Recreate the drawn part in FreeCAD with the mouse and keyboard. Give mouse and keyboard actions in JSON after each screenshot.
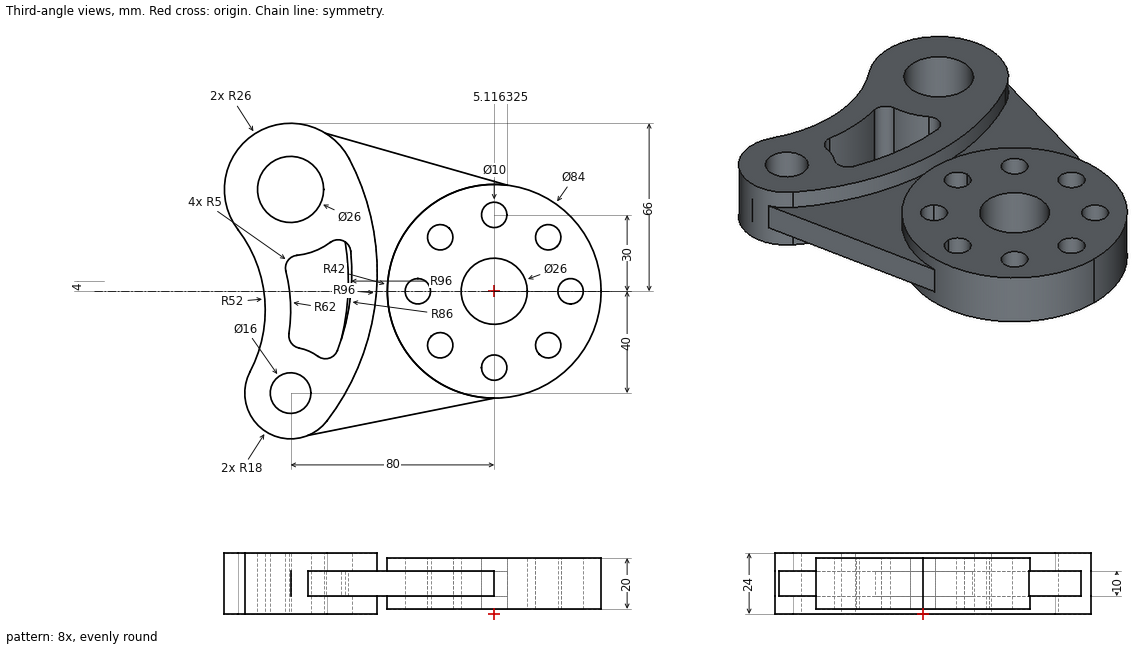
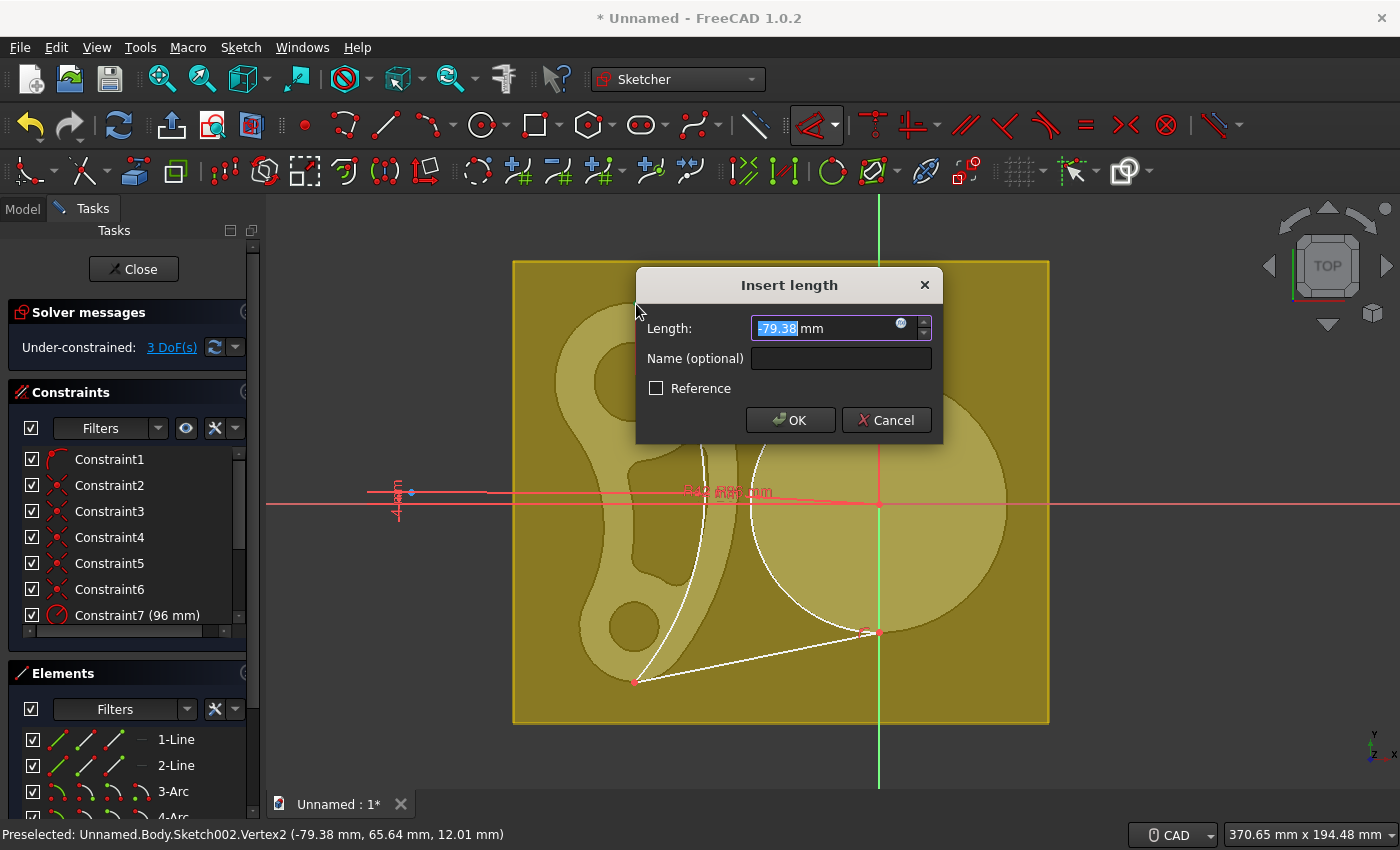
{"action": "type", "text": "-80"}
{"action": "key", "text": "Return"}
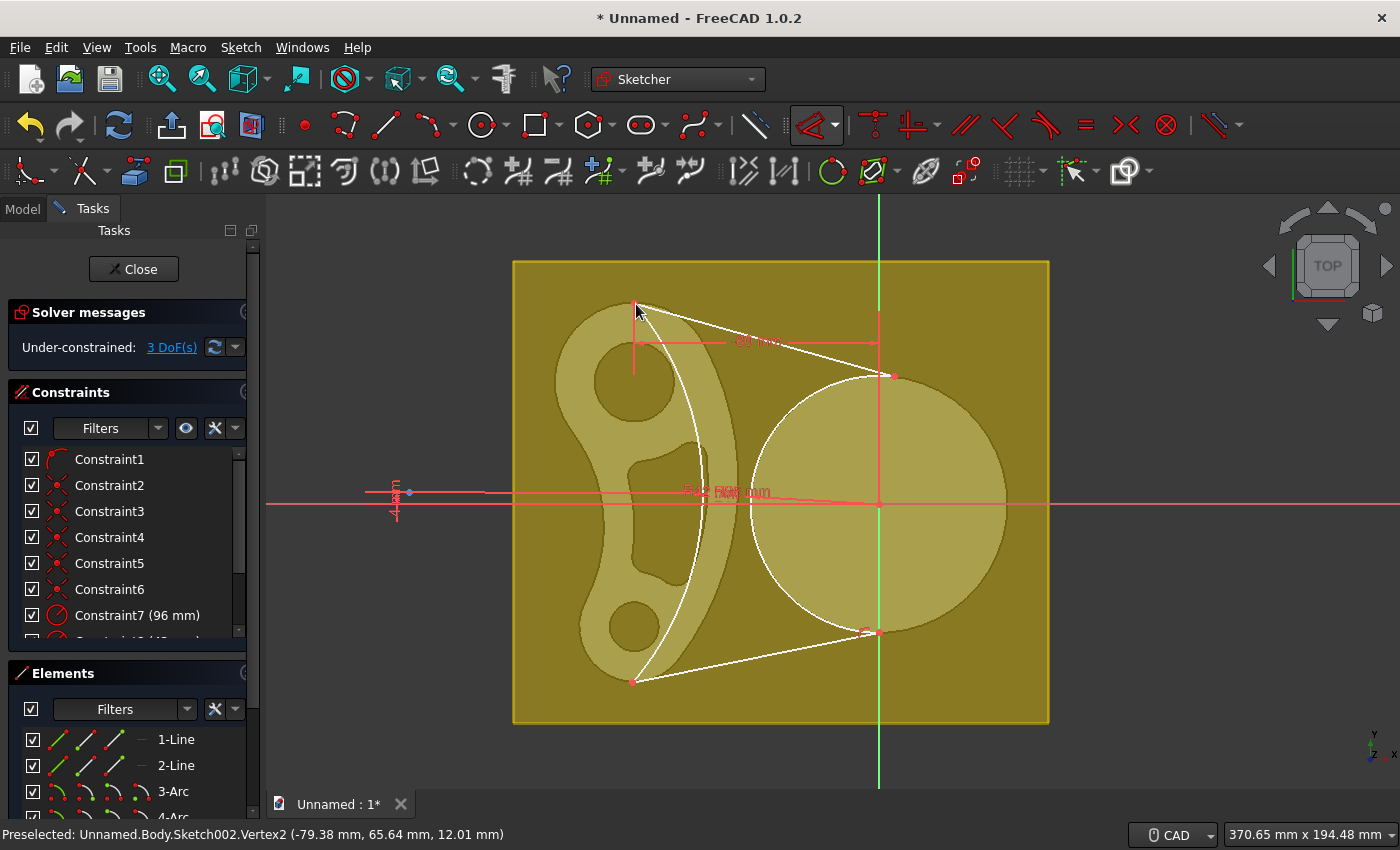
{"action": "left_click", "coordinate": [634, 304]}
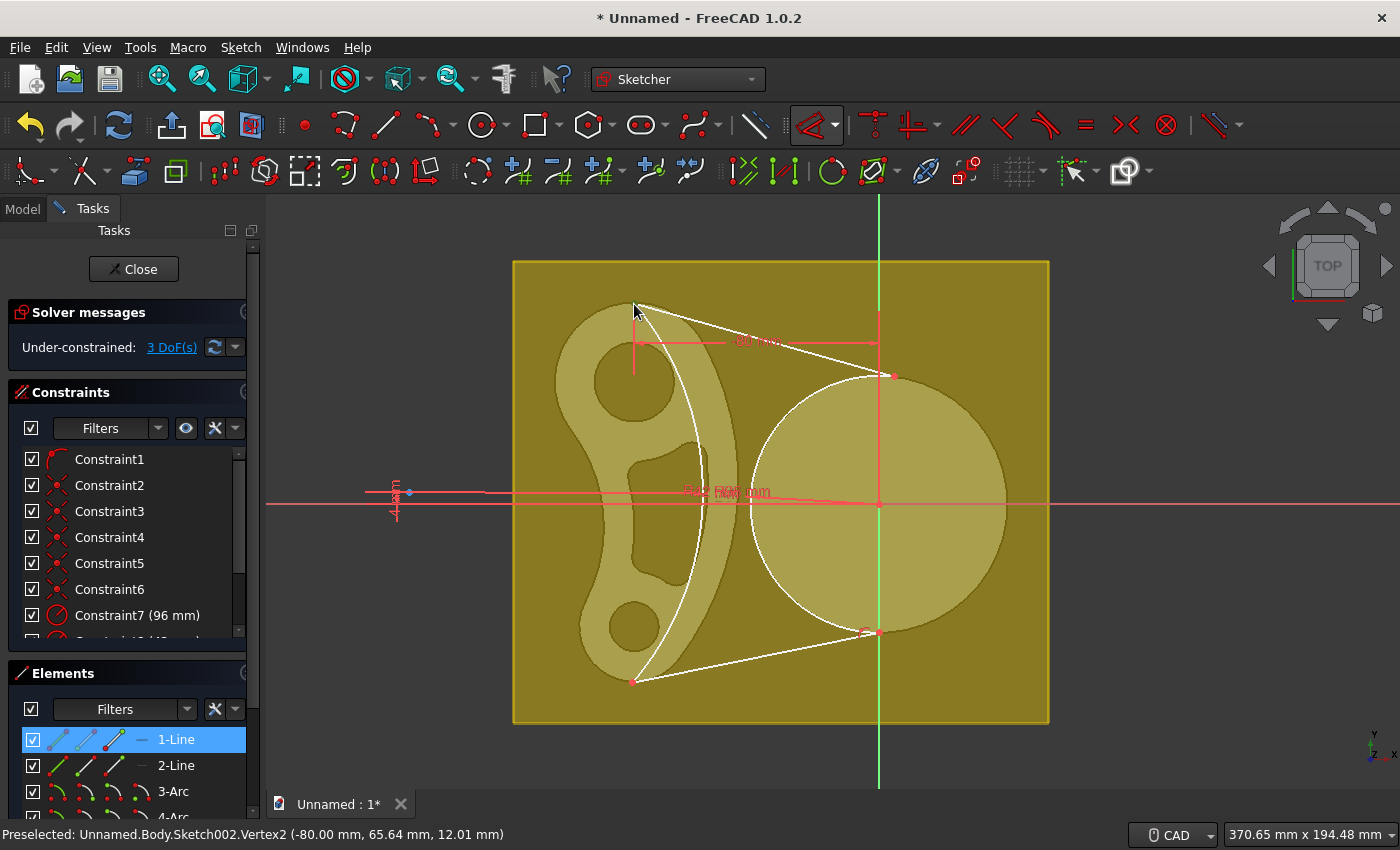
{"action": "key", "text": "i"}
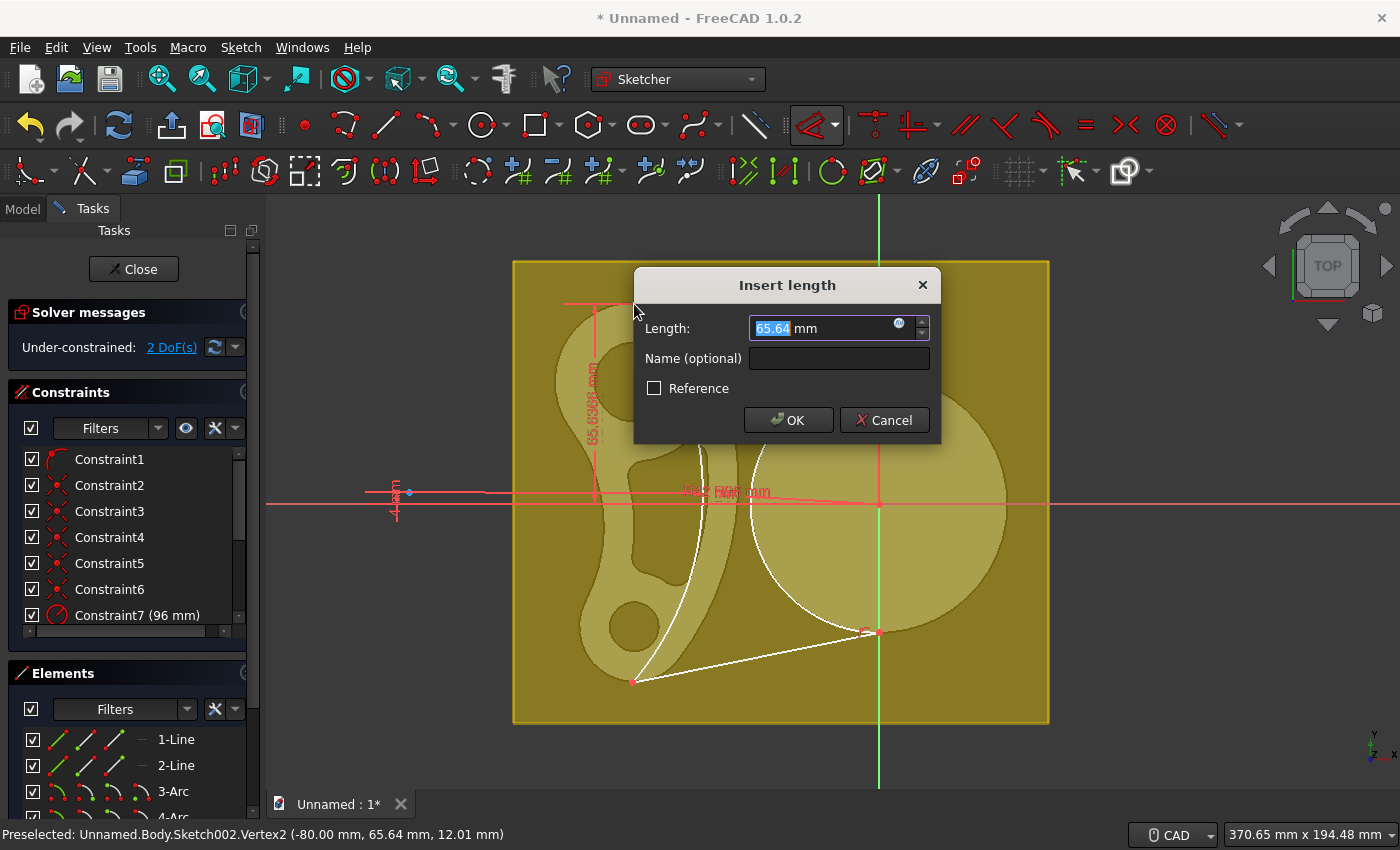
{"action": "type", "text": "66"}
{"action": "key", "text": "Return"}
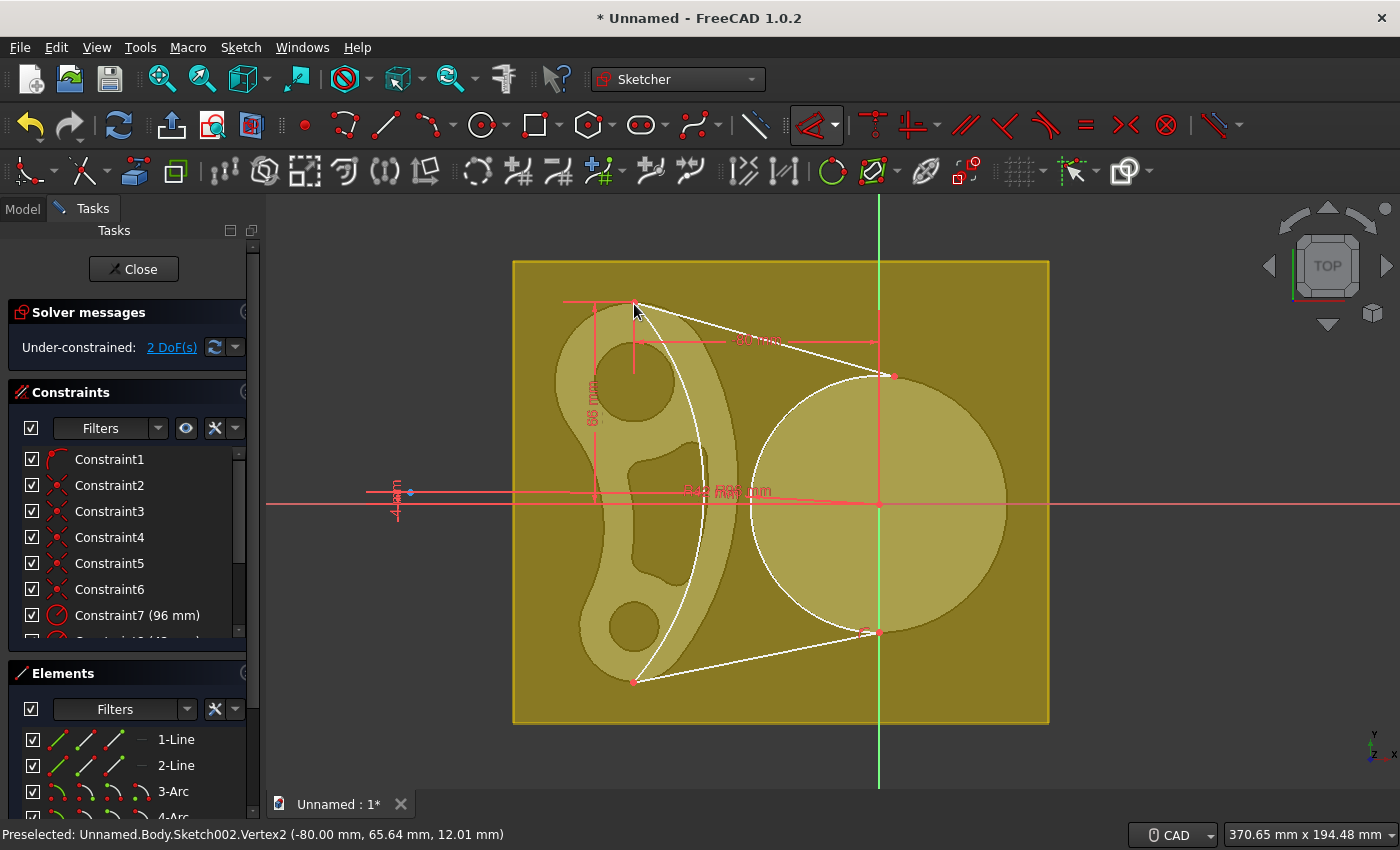
{"action": "left_click", "coordinate": [633, 683]}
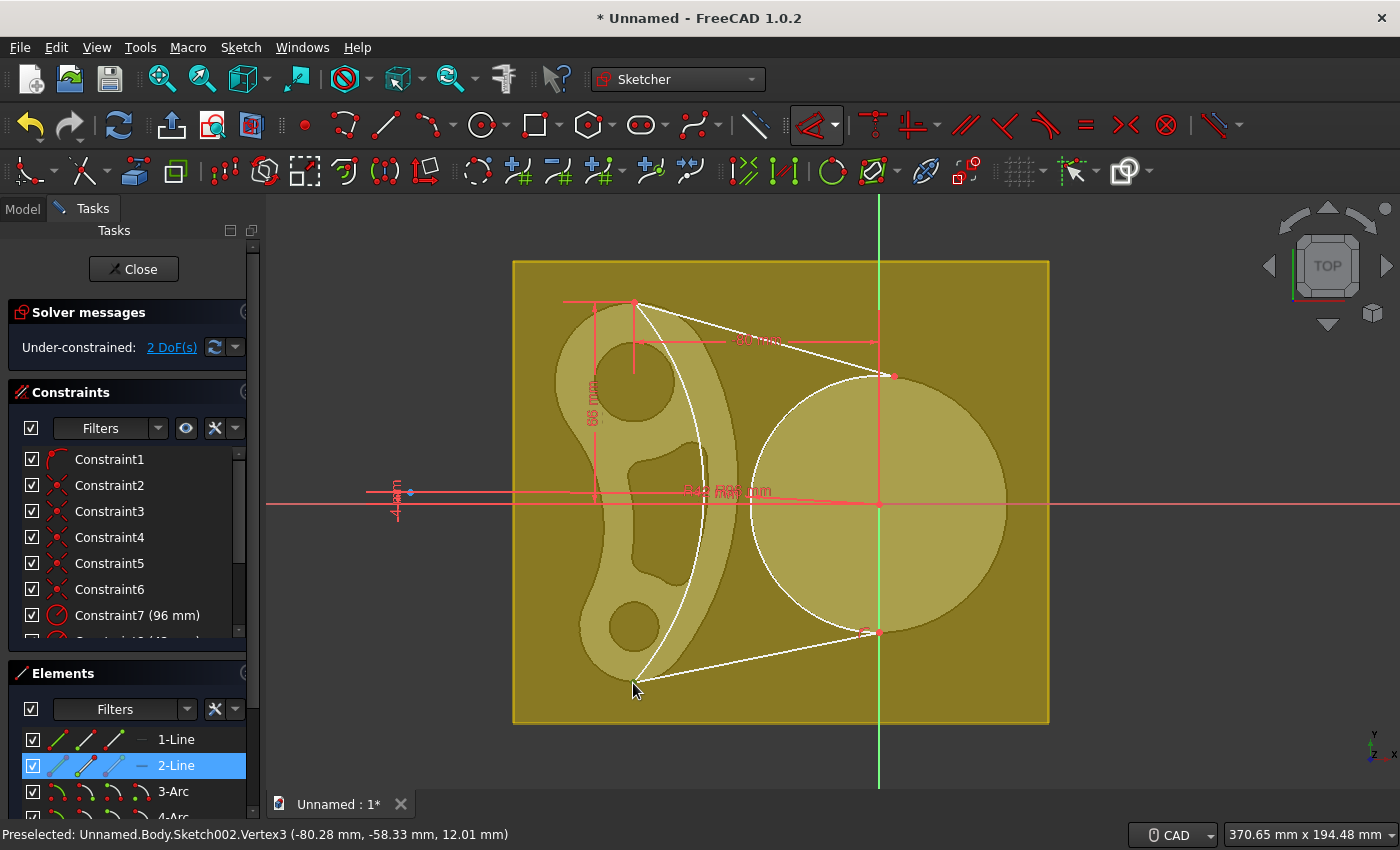
{"action": "key", "text": "l"}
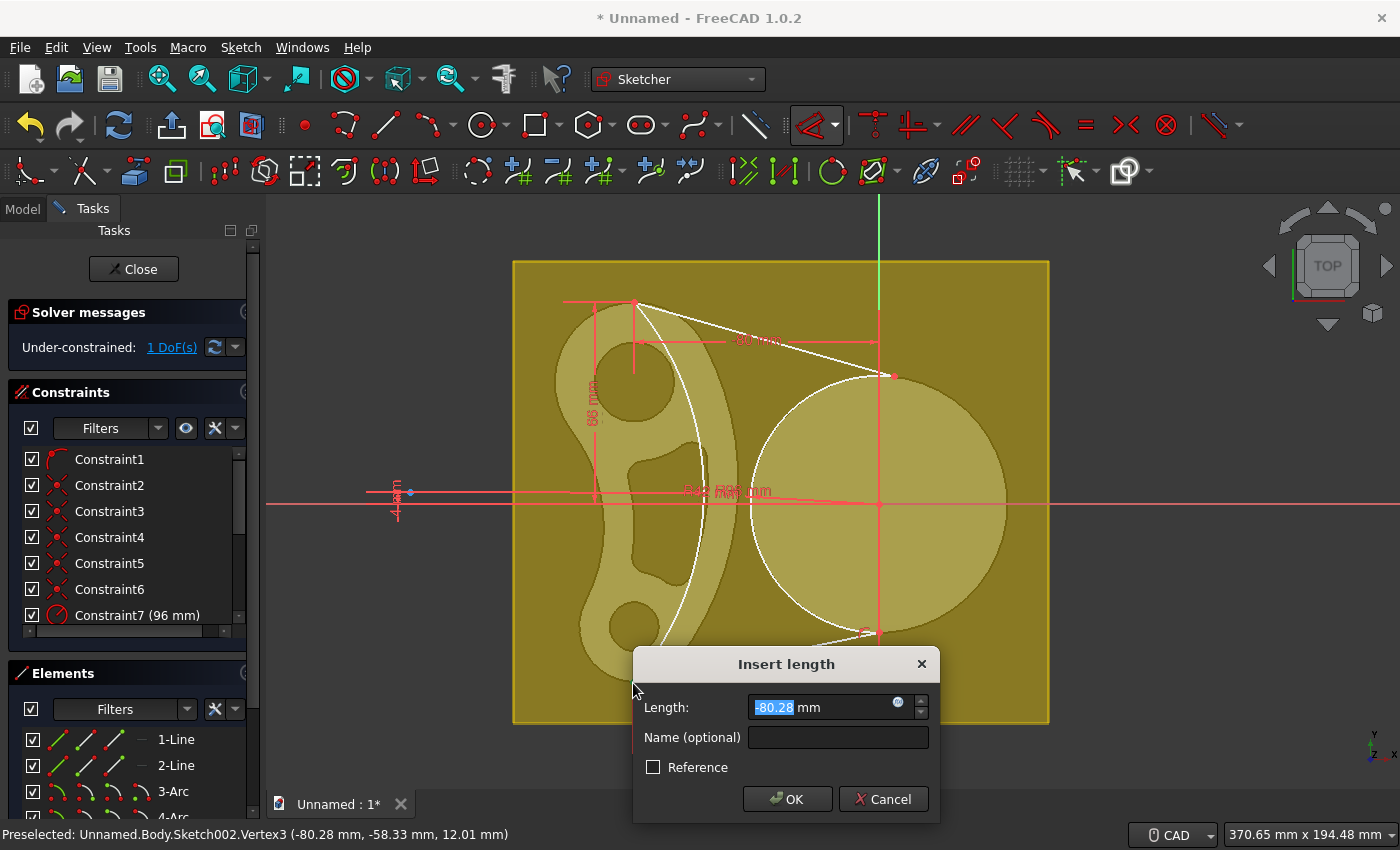
{"action": "type", "text": "-80"}
{"action": "key", "text": "Return"}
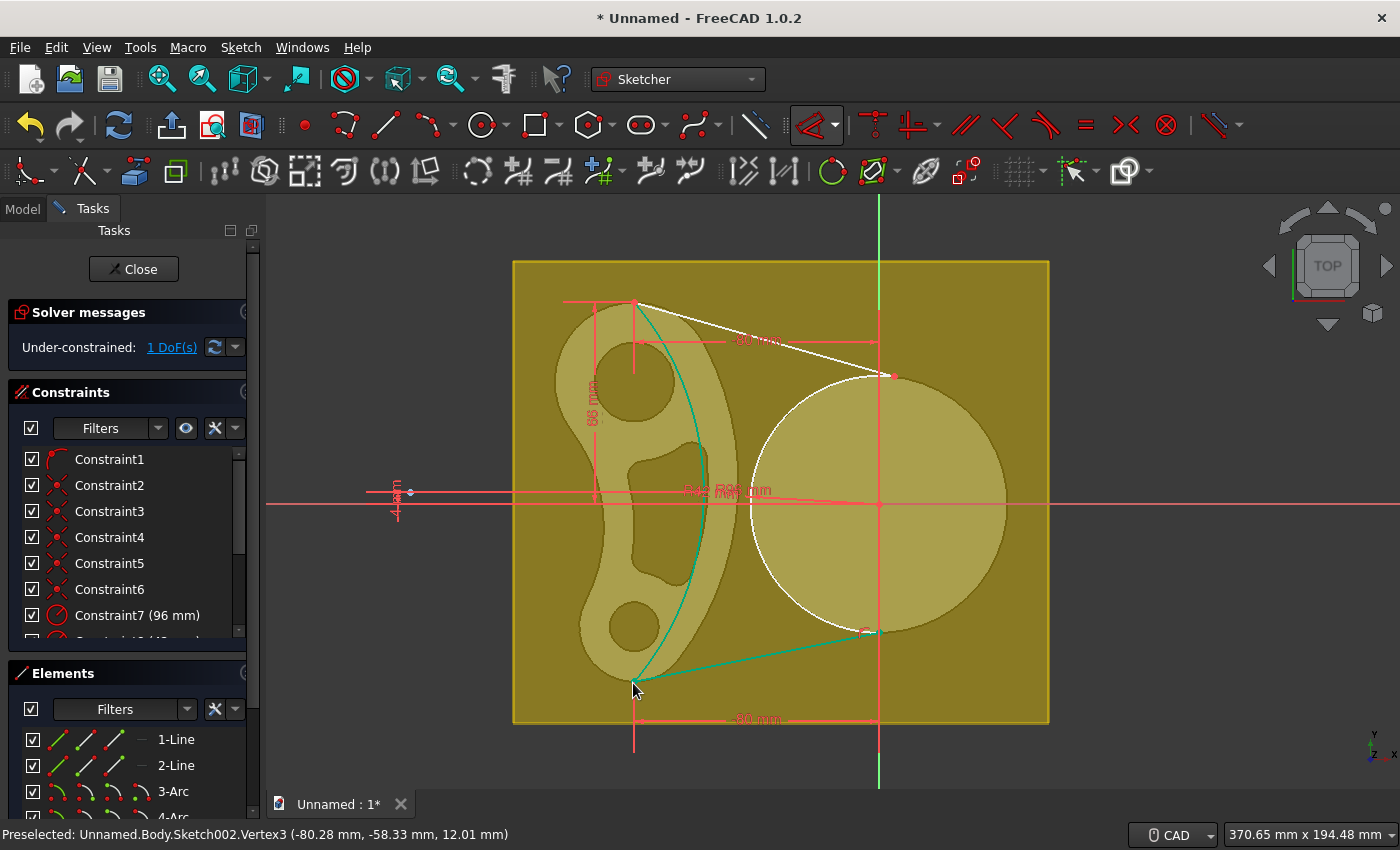
{"action": "scroll", "coordinate": [894, 377], "scroll_direction": "up", "scroll_amount": 5}